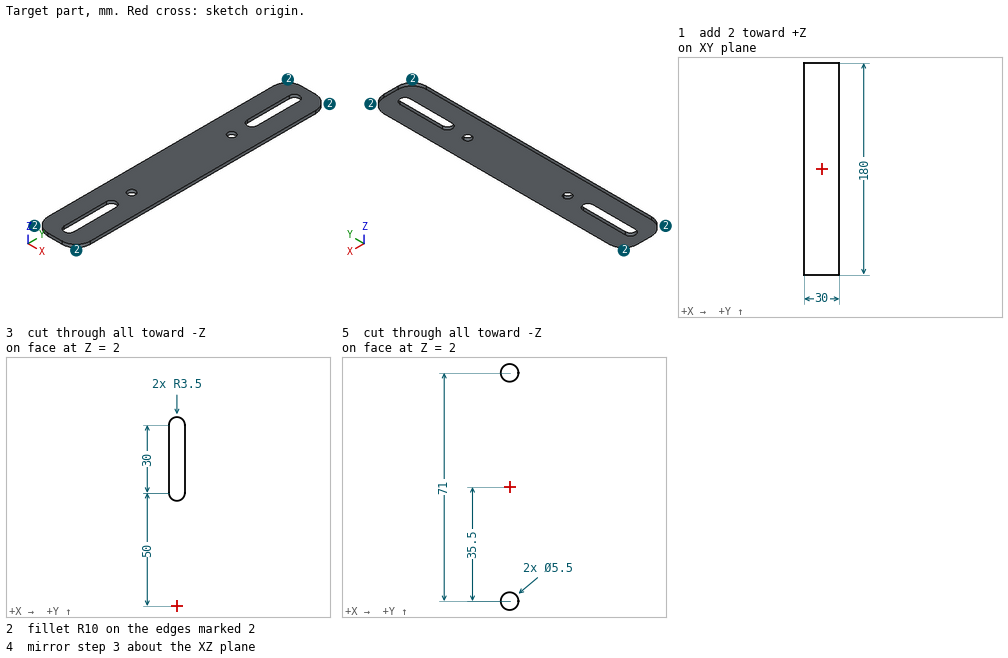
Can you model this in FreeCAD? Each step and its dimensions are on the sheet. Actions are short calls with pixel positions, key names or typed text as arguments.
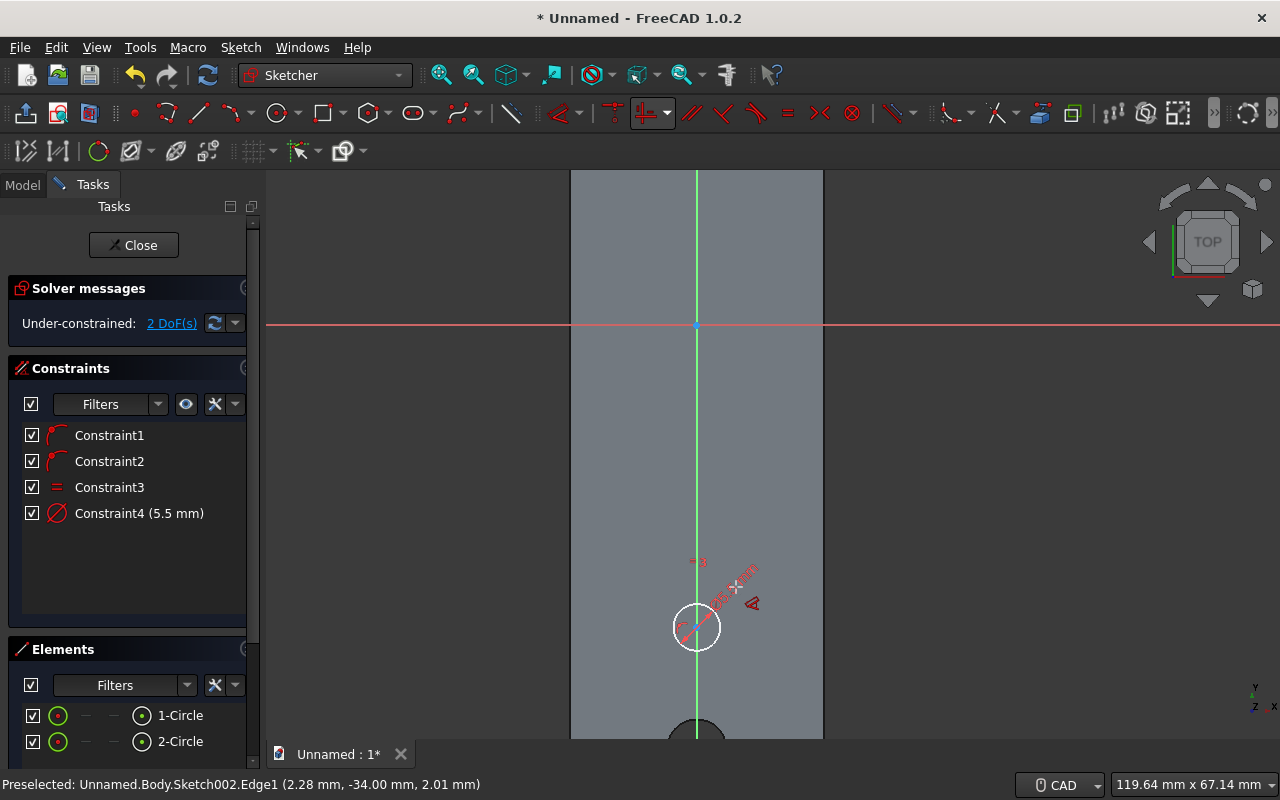
click(697, 627)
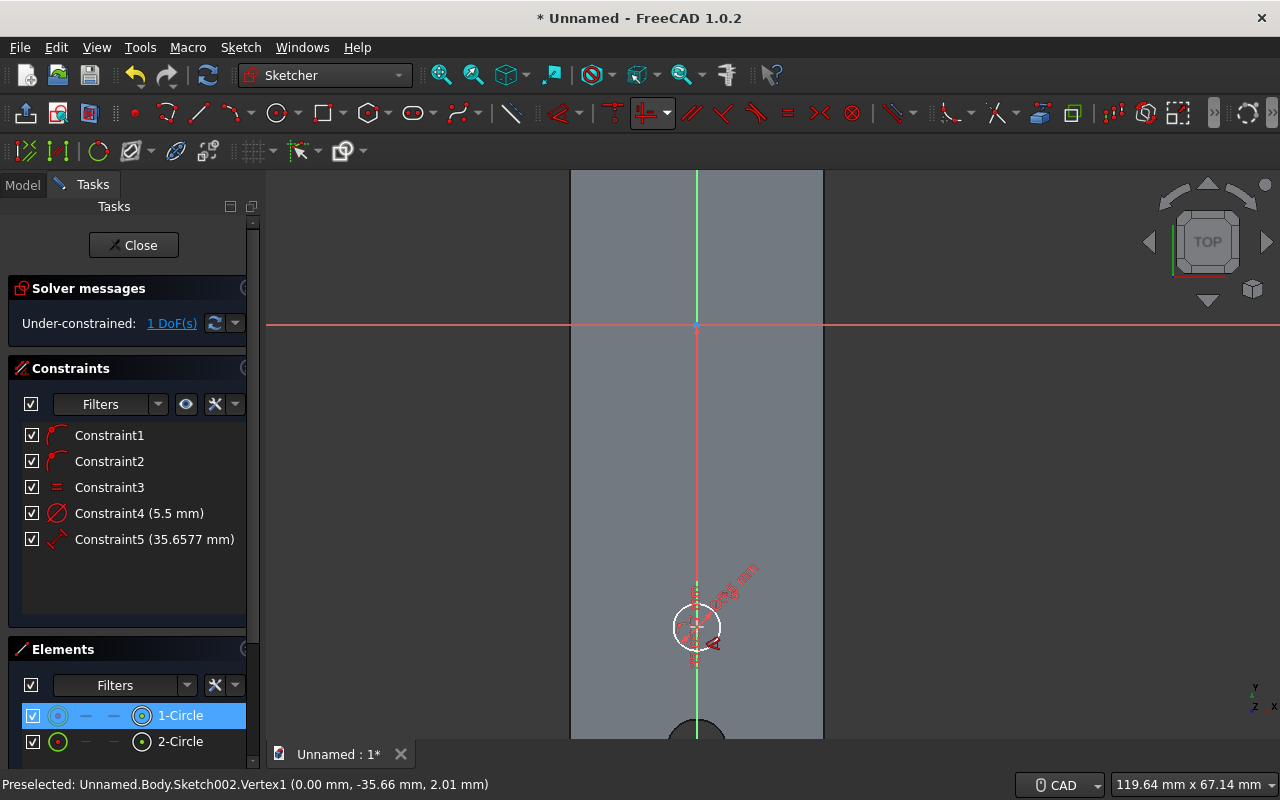
scroll(714, 612, down, 3)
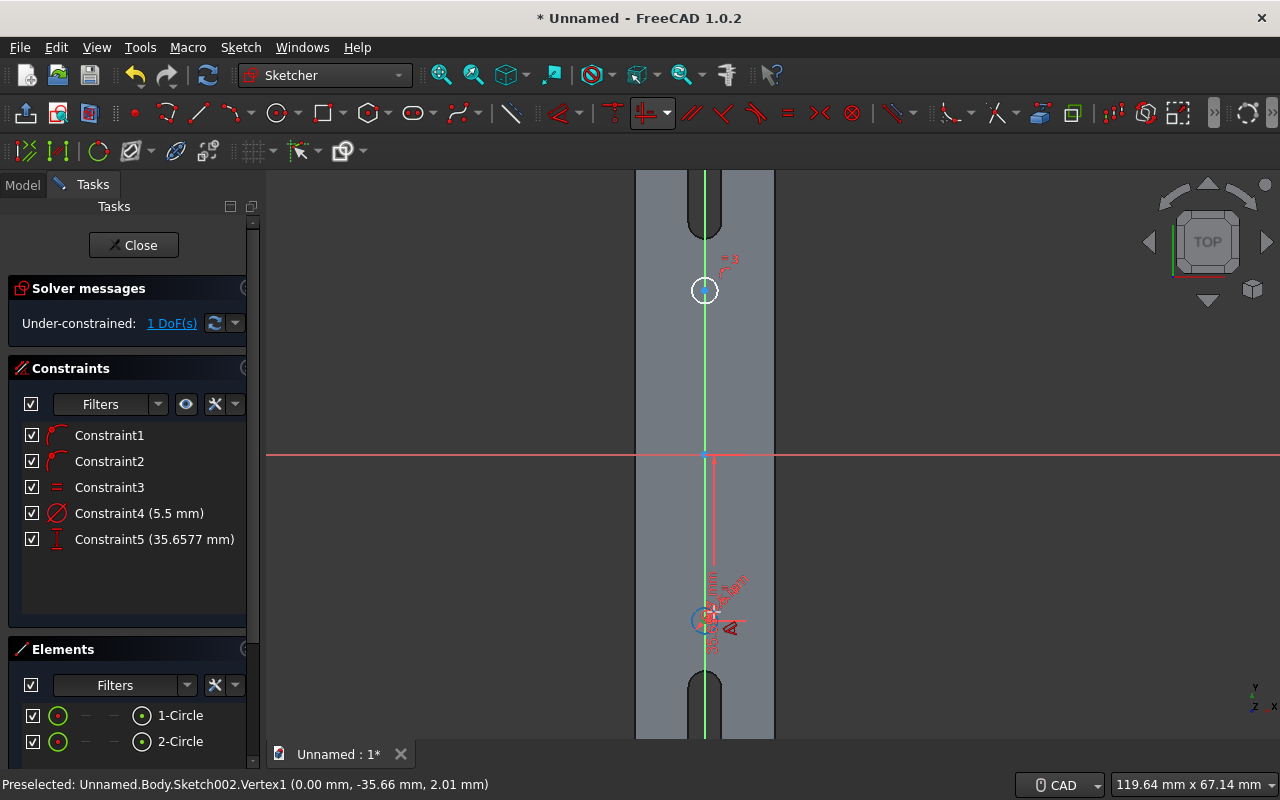
click(705, 291)
click(739, 380)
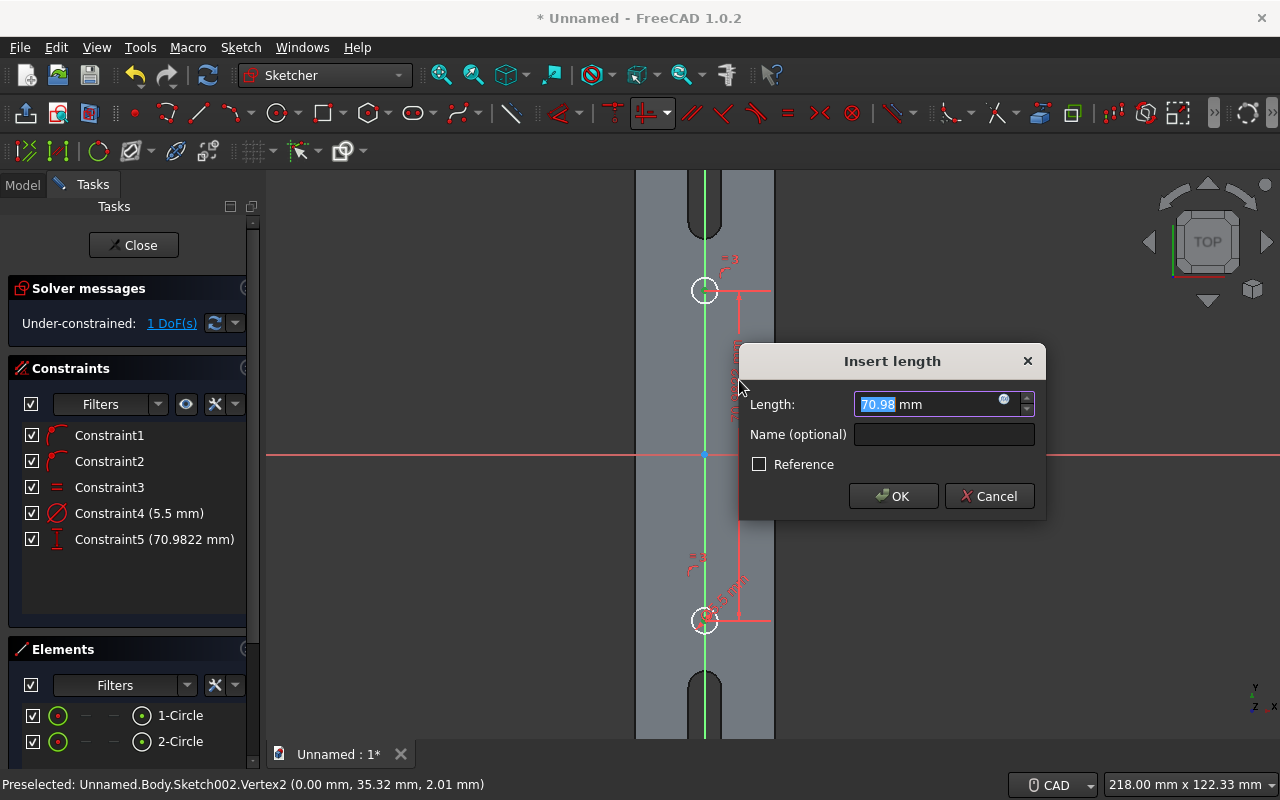
text(71)
key(Return)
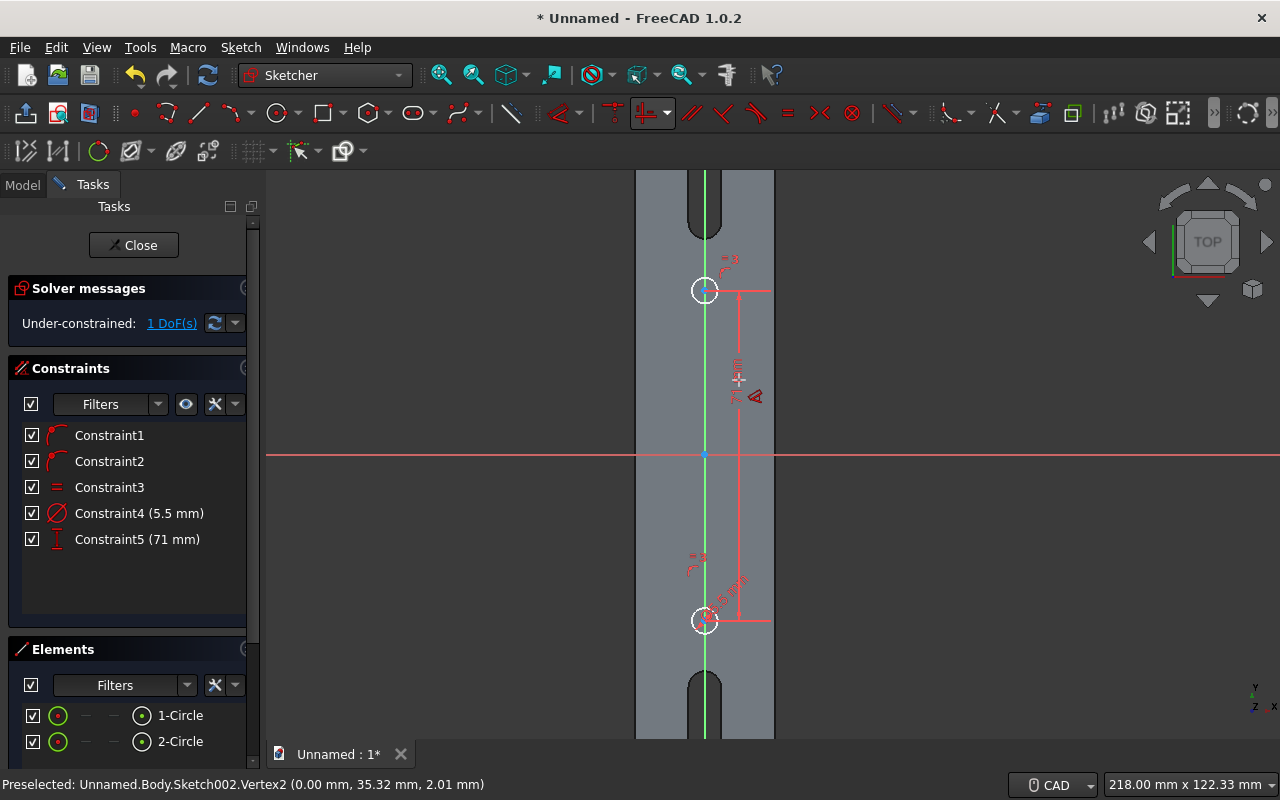
click(705, 621)
click(739, 538)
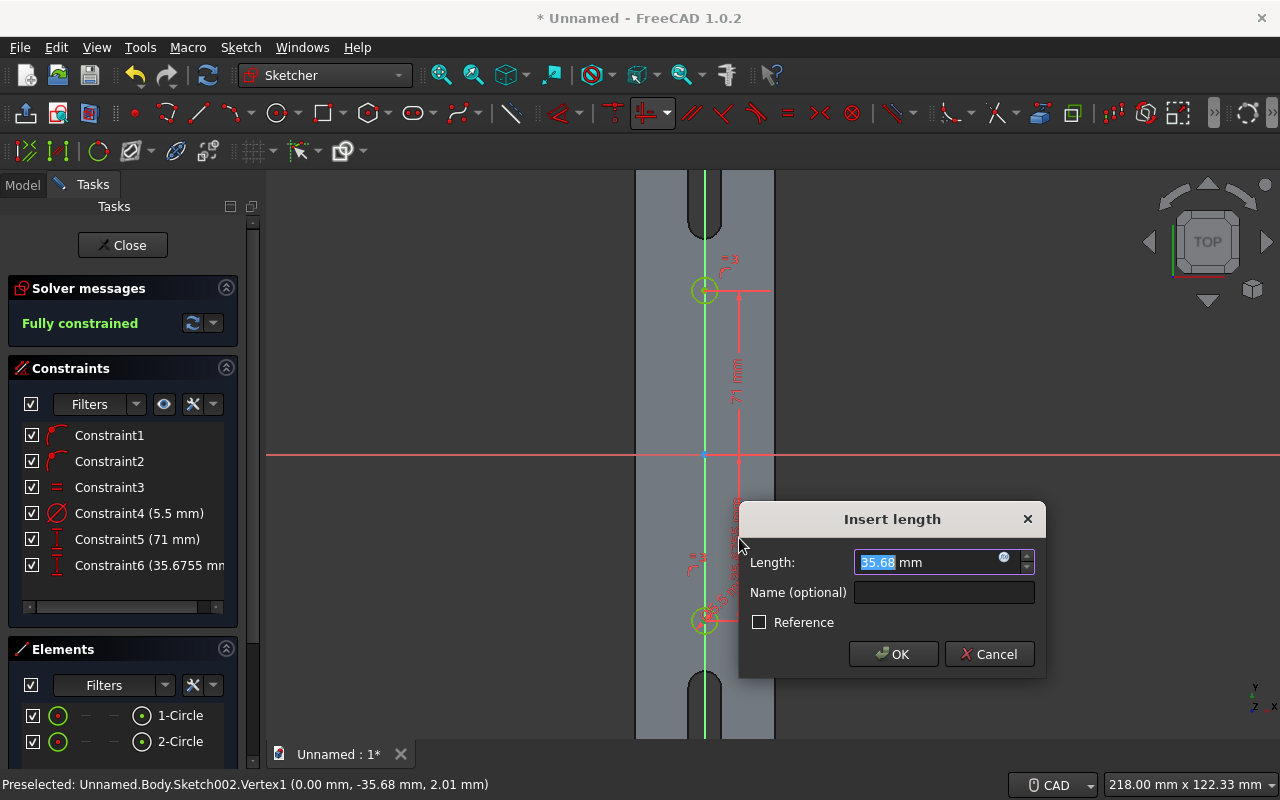
text(35.5)
key(Return)
key(Escape)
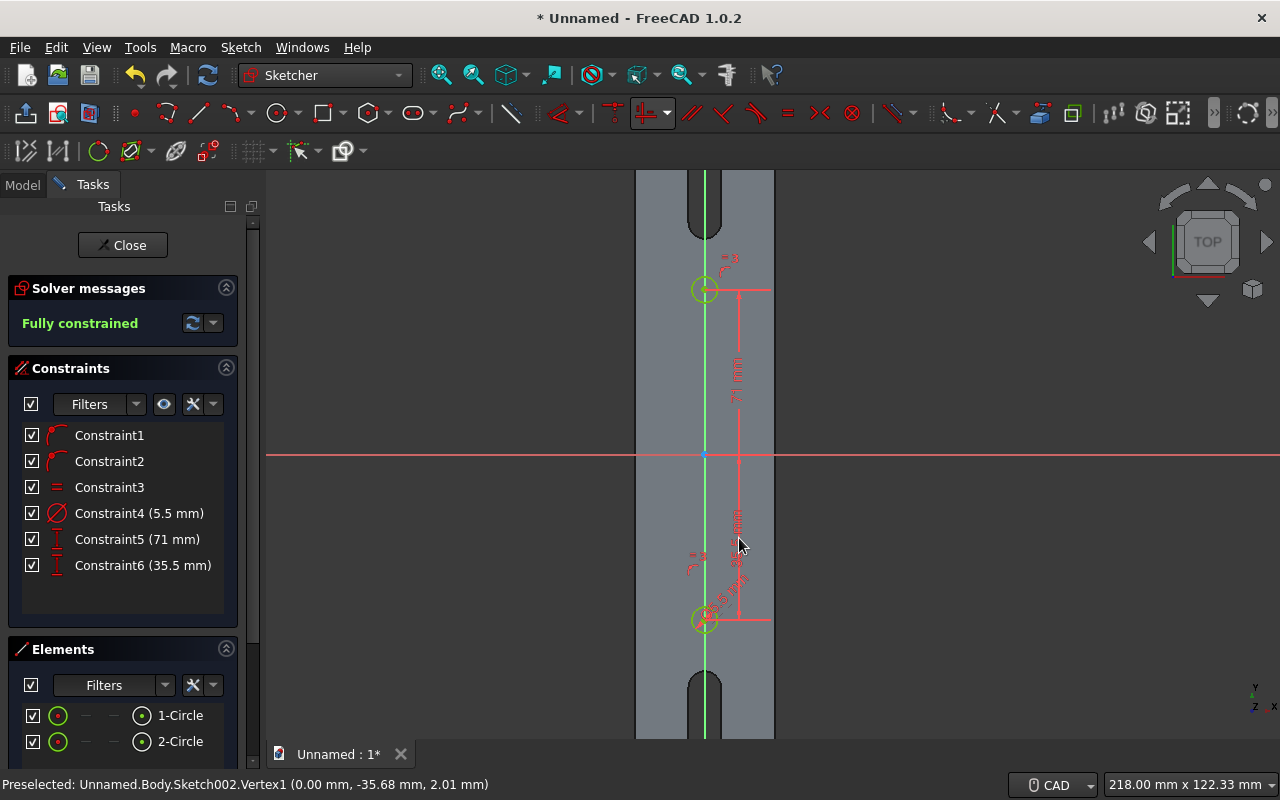
click(123, 245)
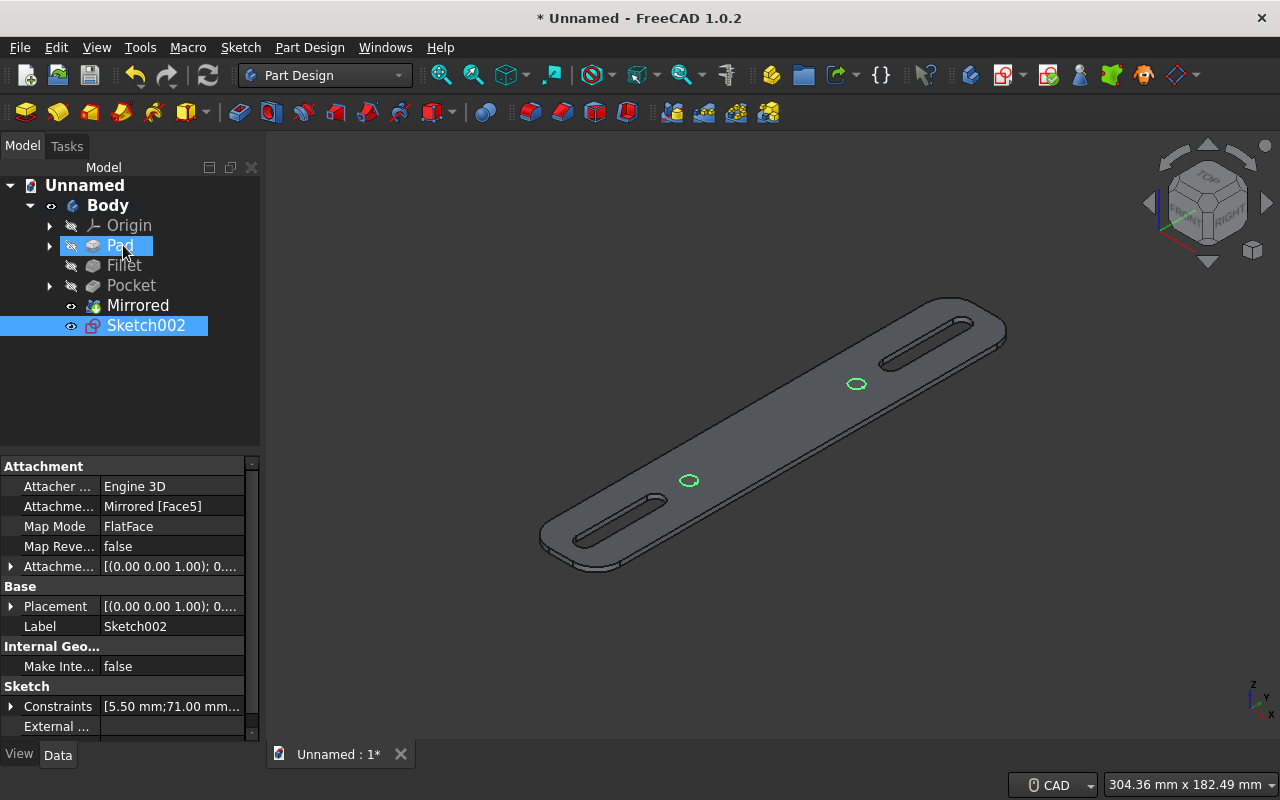
click(240, 112)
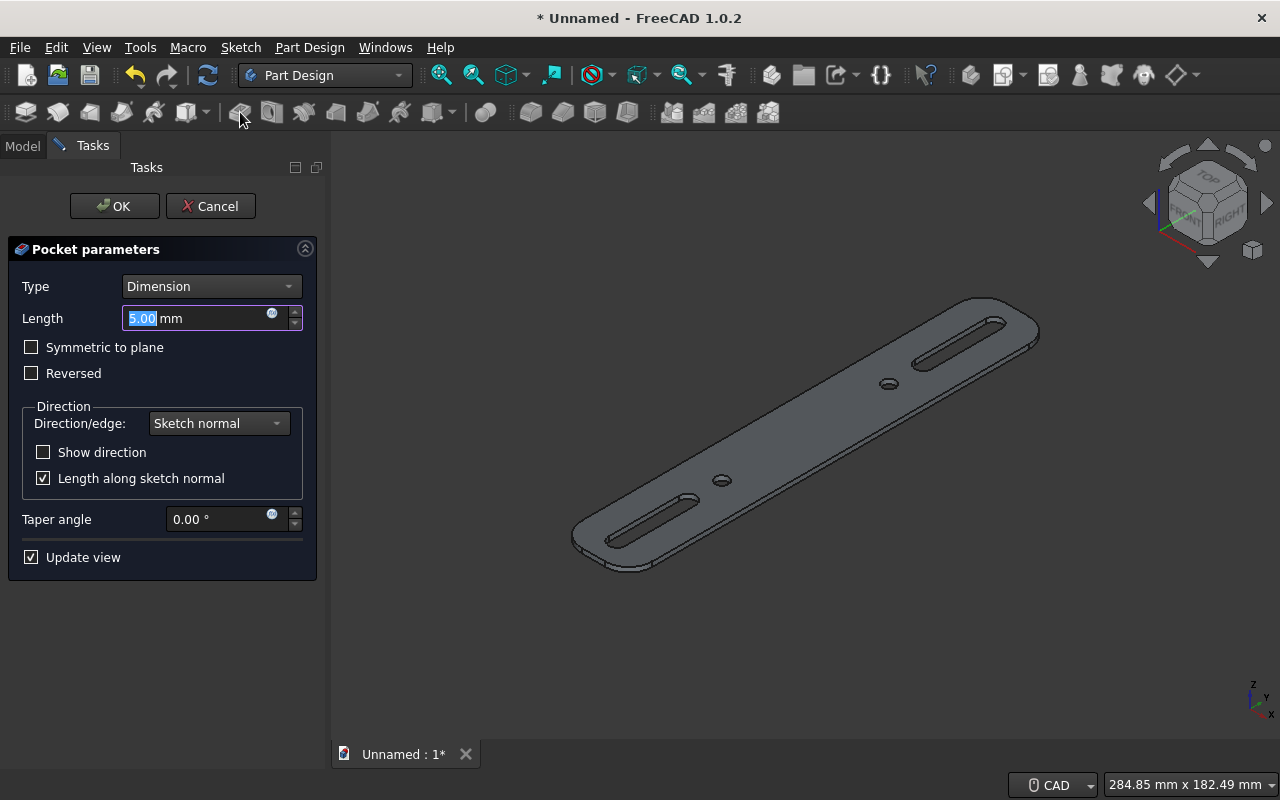
click(212, 286)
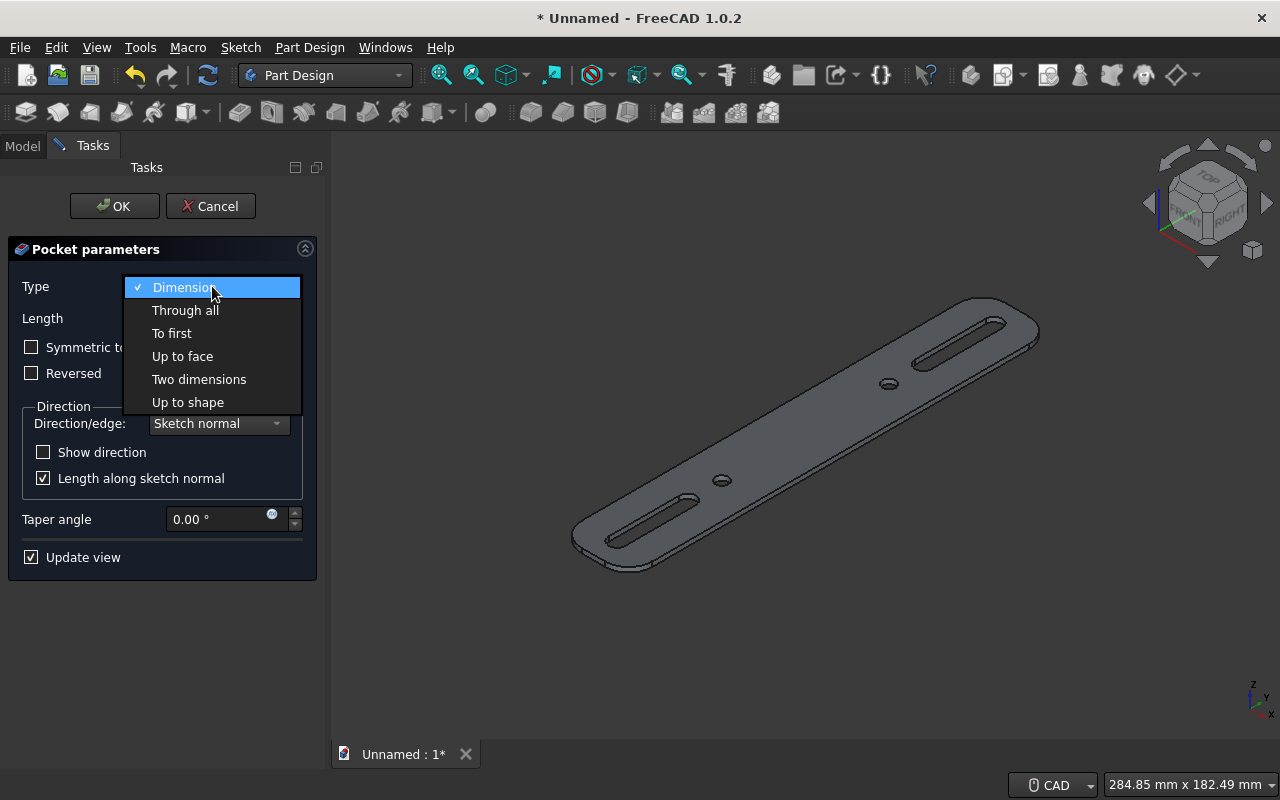
click(212, 310)